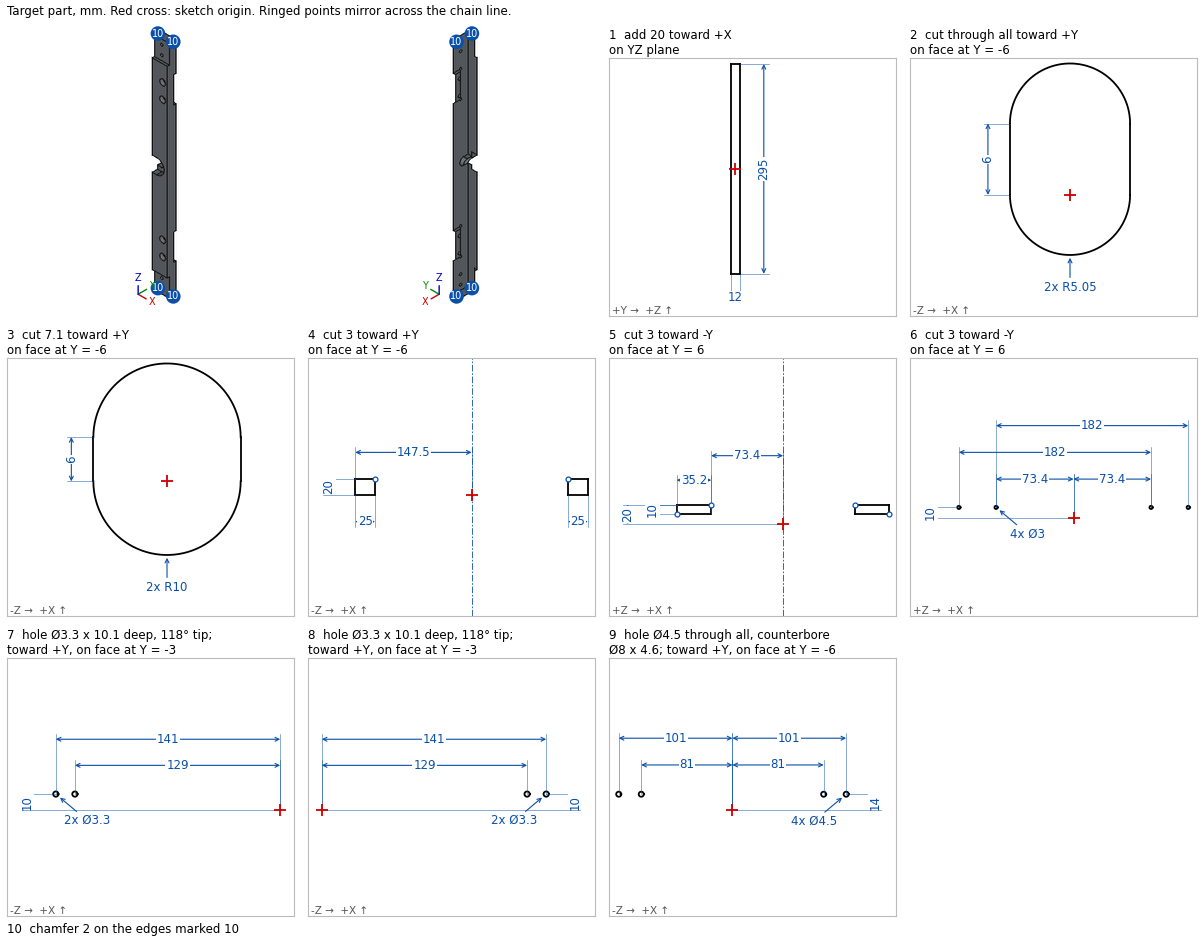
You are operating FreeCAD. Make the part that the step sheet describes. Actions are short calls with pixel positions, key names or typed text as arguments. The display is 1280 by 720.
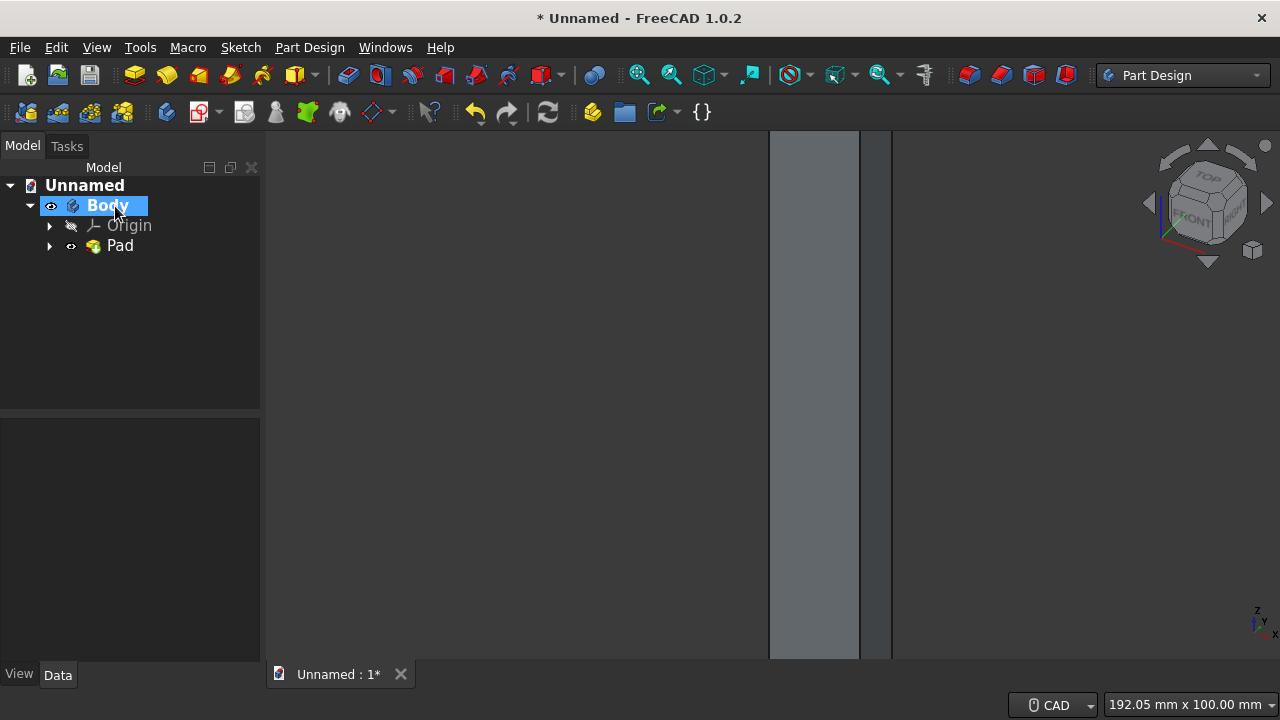
click(640, 76)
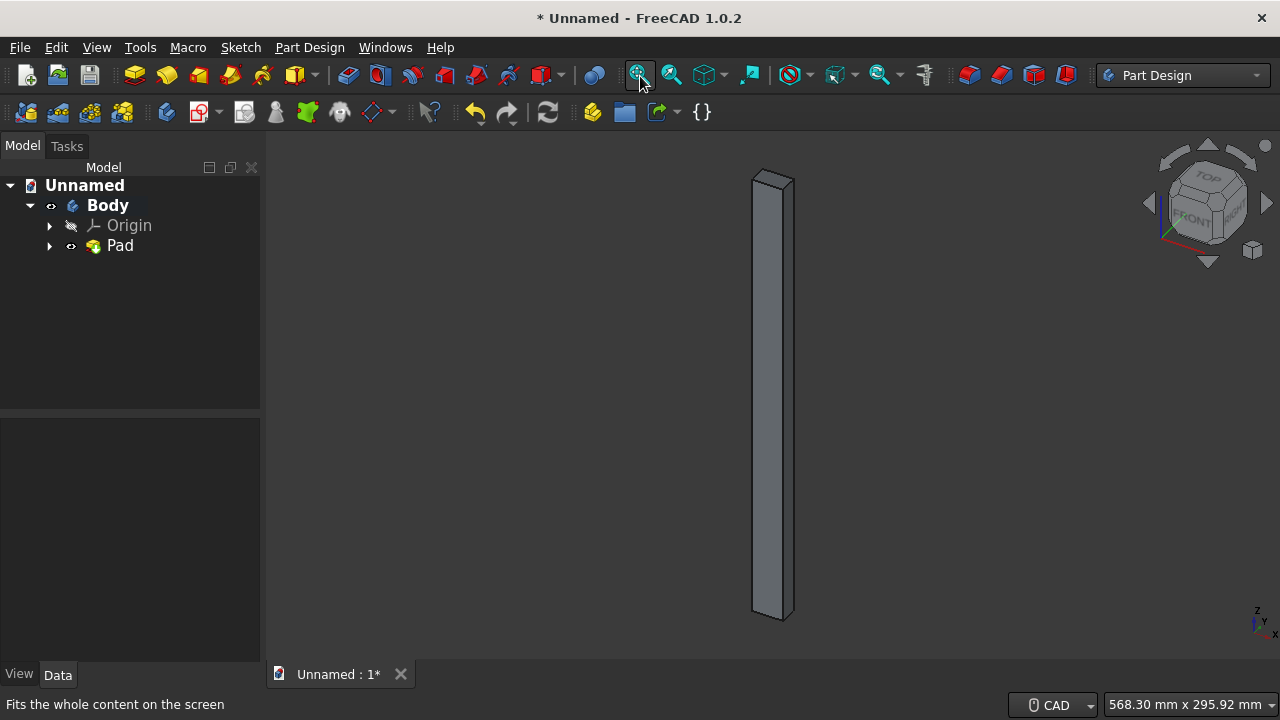
click(768, 584)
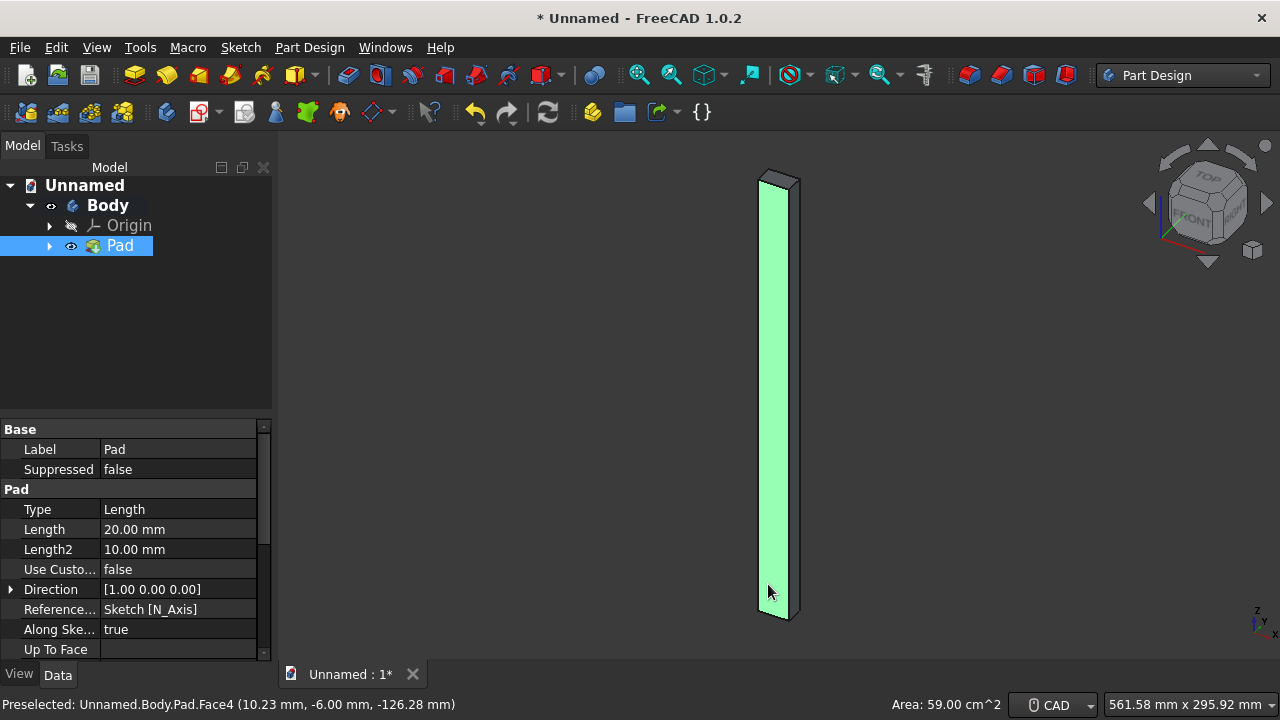
click(200, 112)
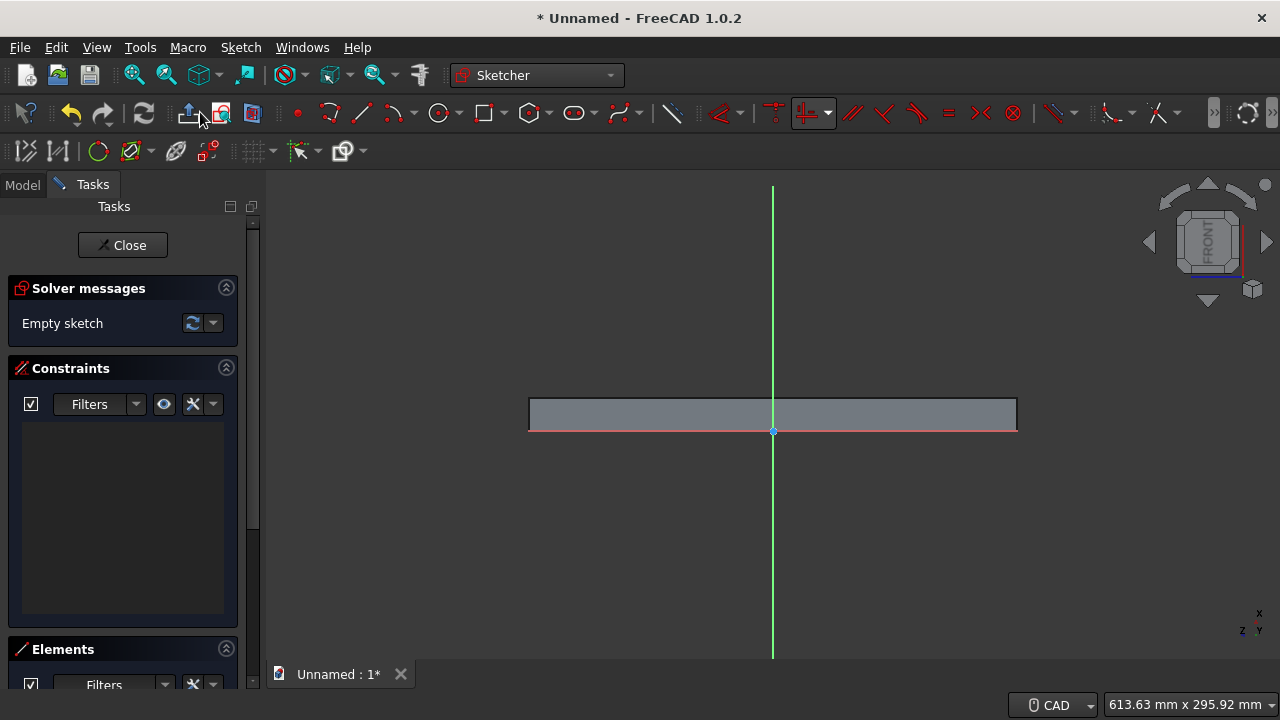
scroll(780, 427, up, 12)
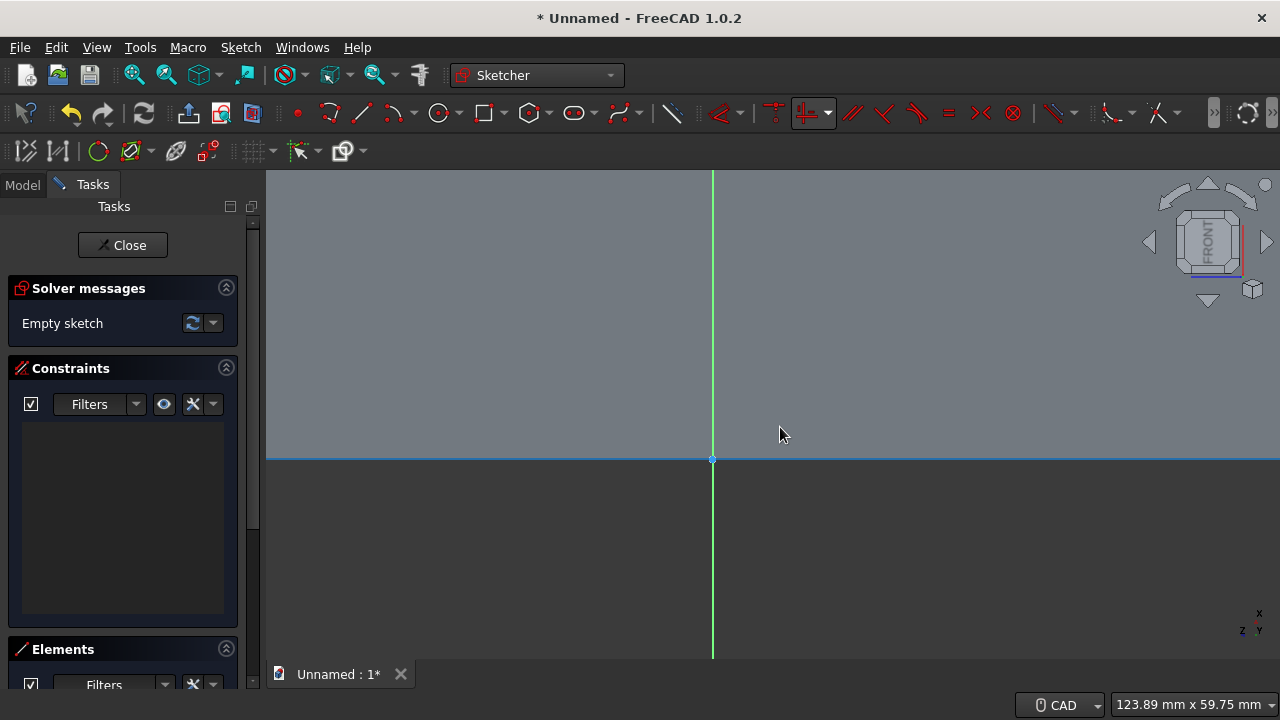
click(574, 114)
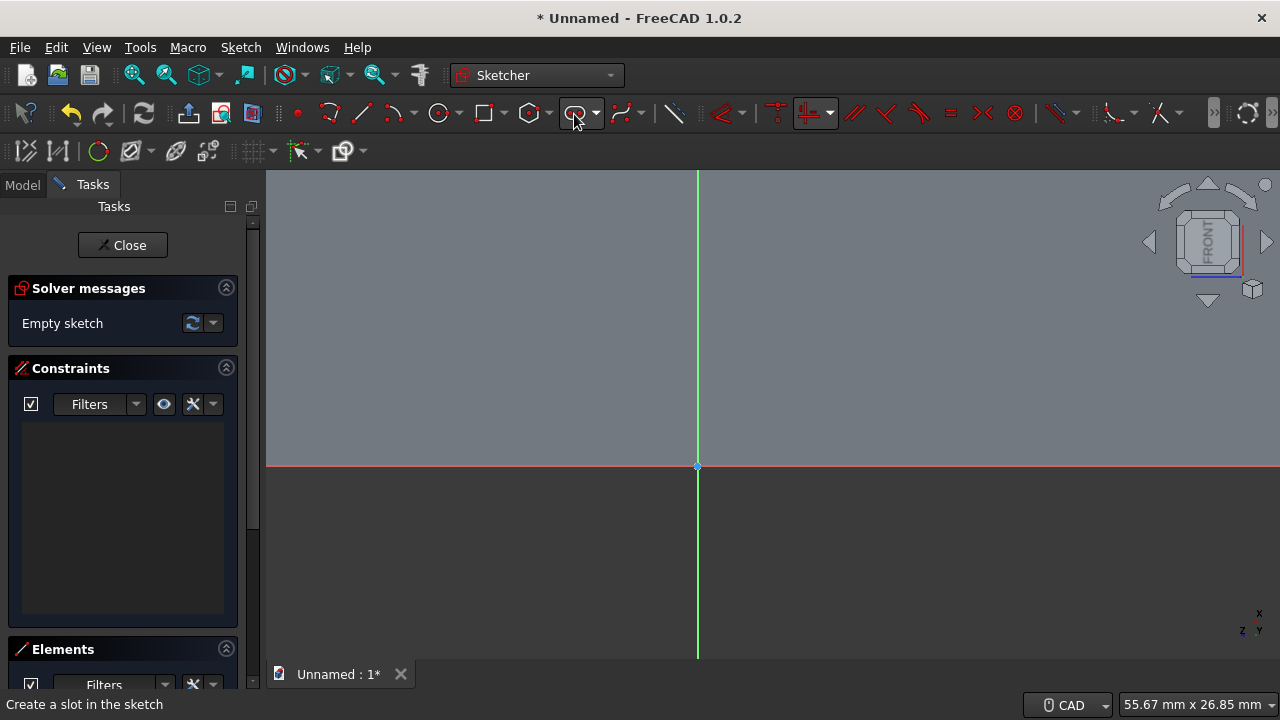
click(698, 466)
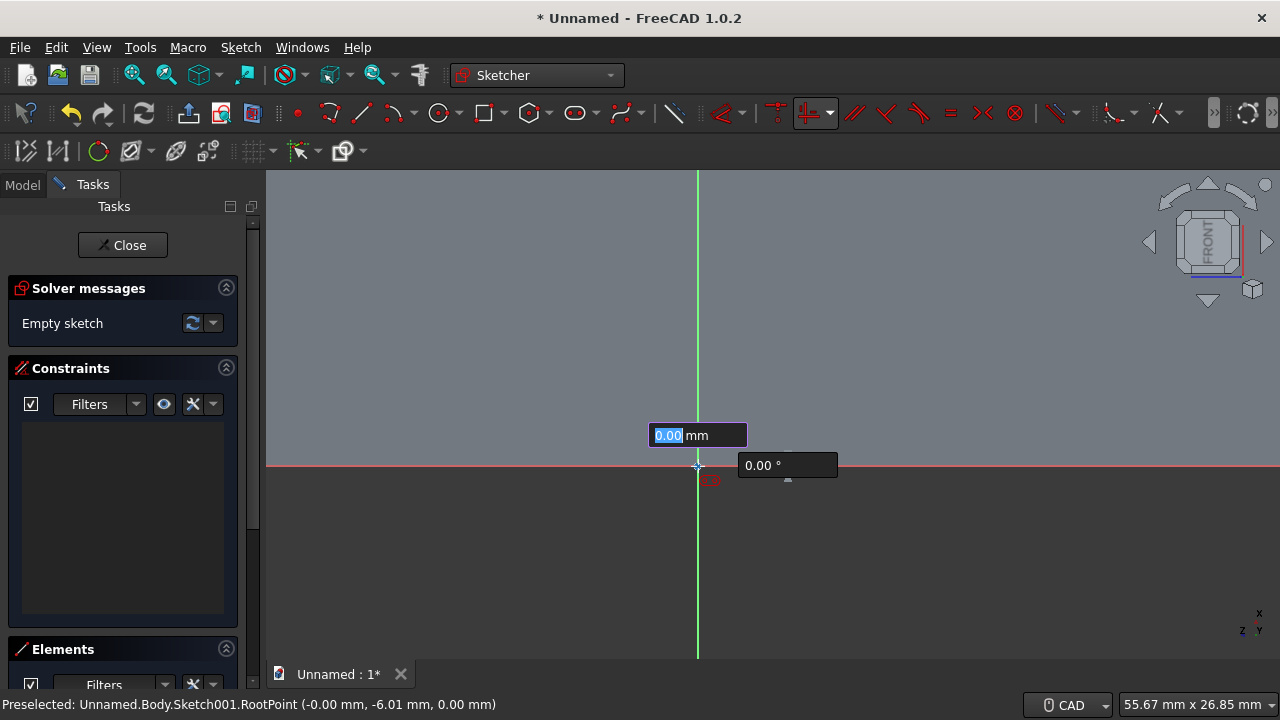
click(707, 357)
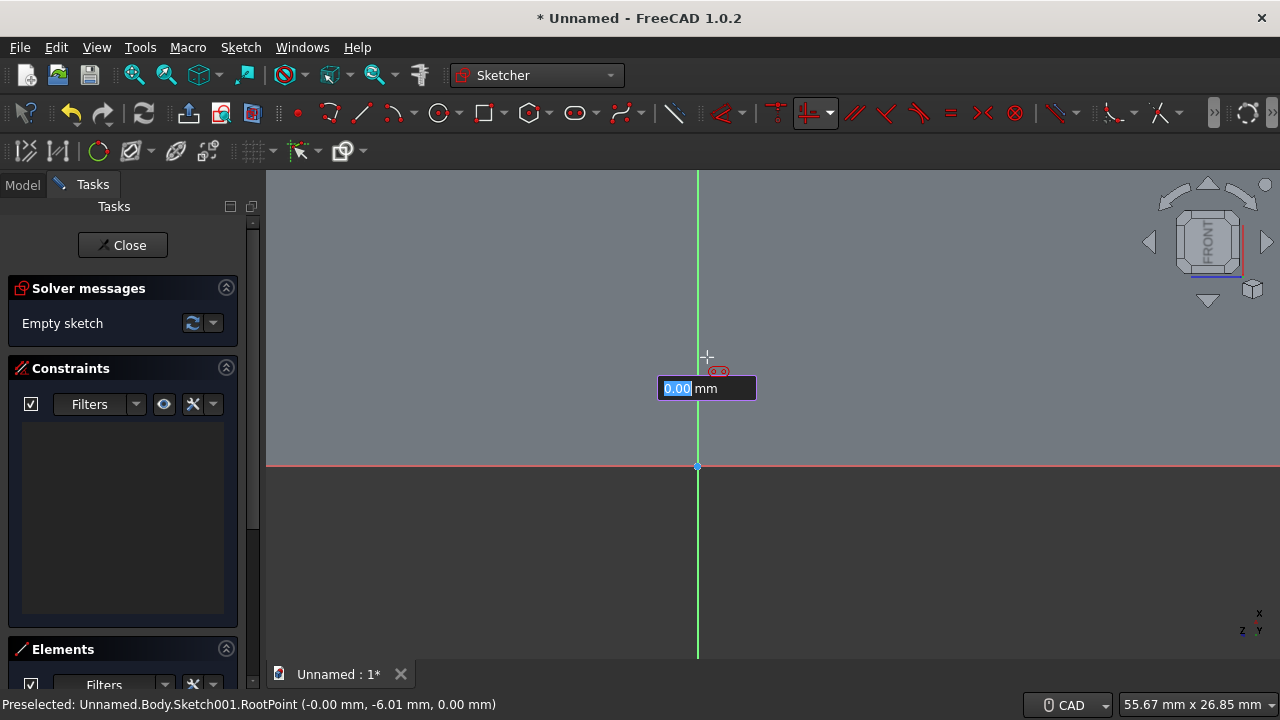
click(606, 411)
key(Escape)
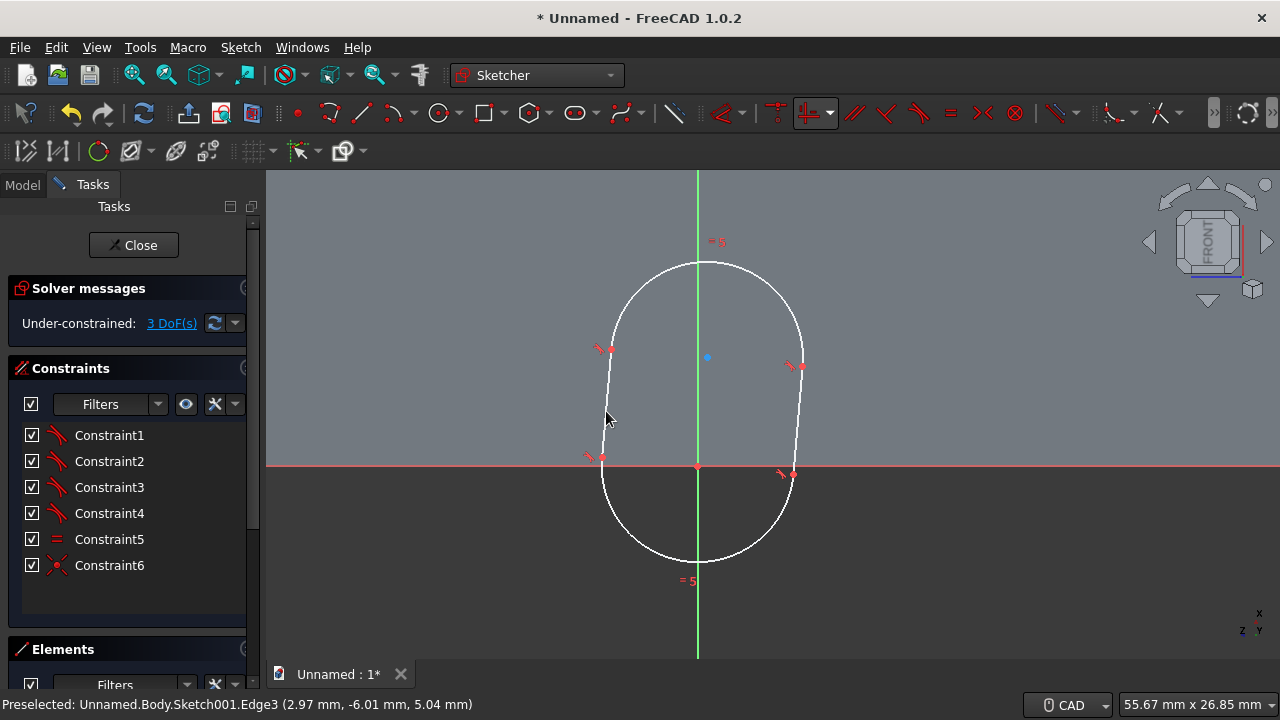
click(605, 425)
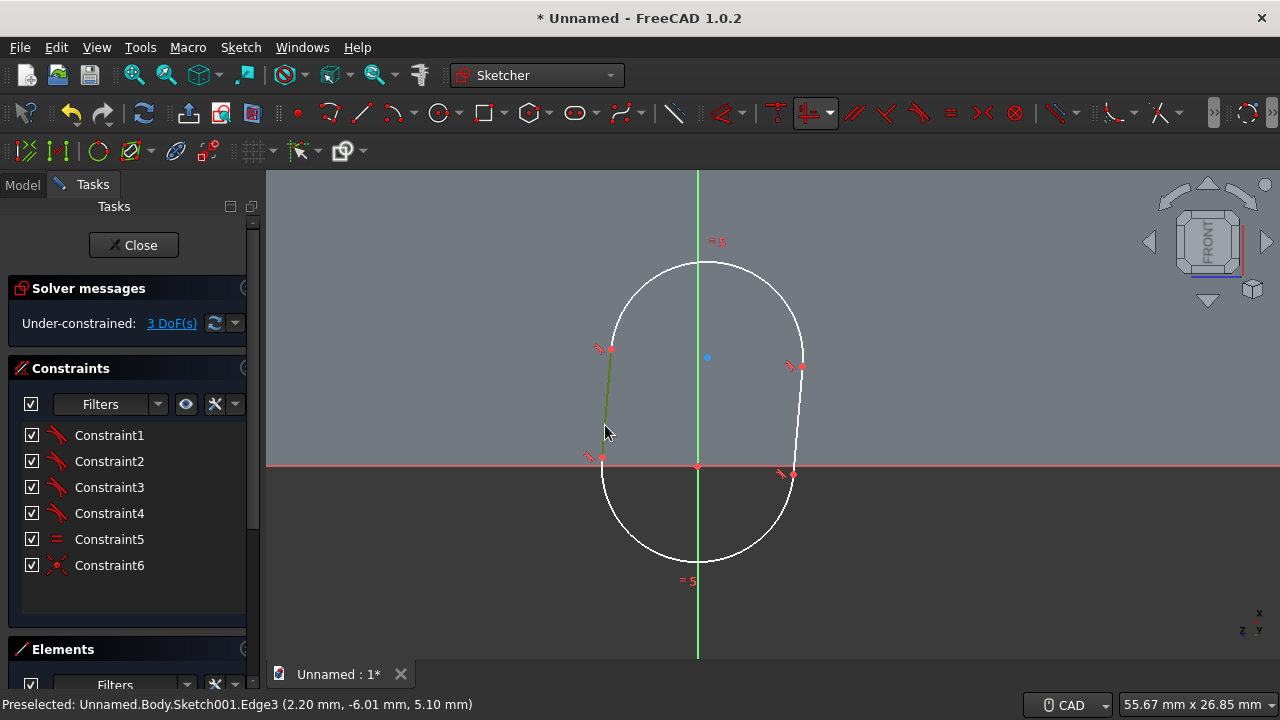
click(832, 114)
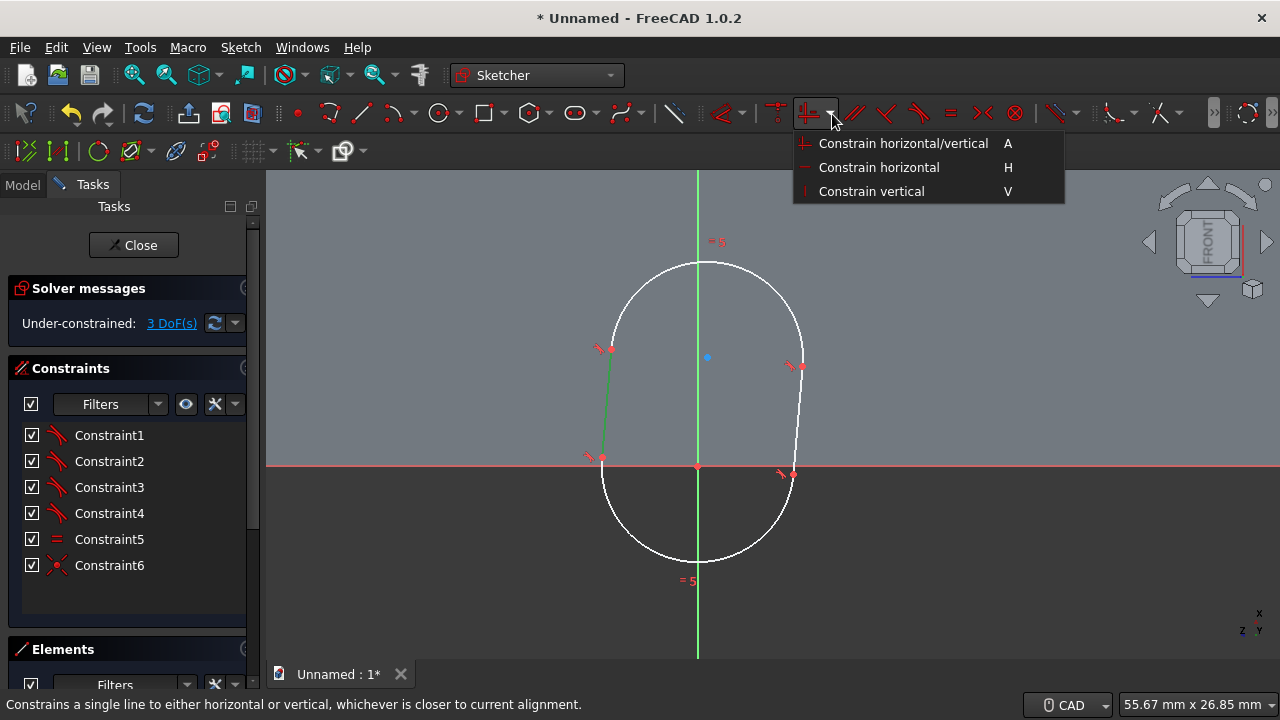
click(929, 191)